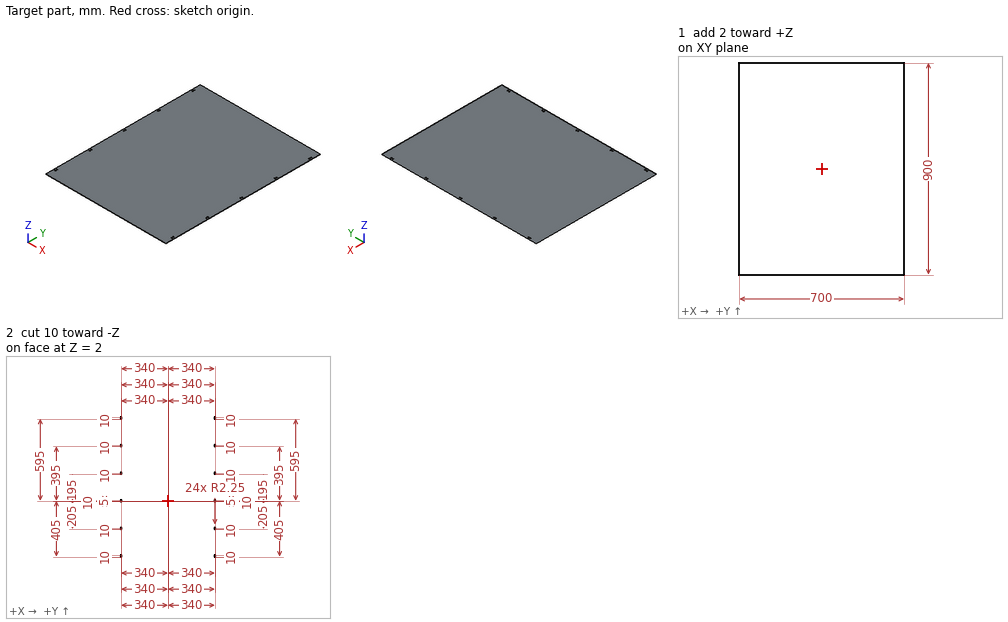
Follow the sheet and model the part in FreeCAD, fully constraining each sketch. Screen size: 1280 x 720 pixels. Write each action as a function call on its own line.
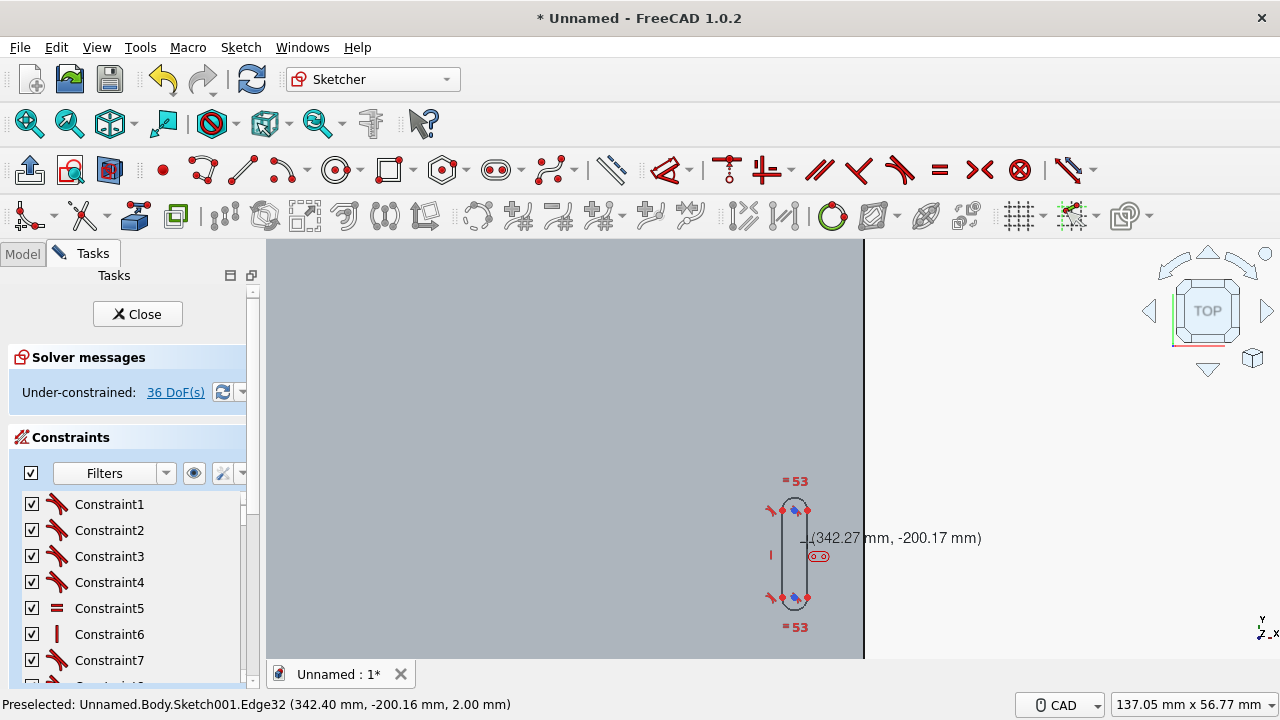
scroll(808, 539, down, 16)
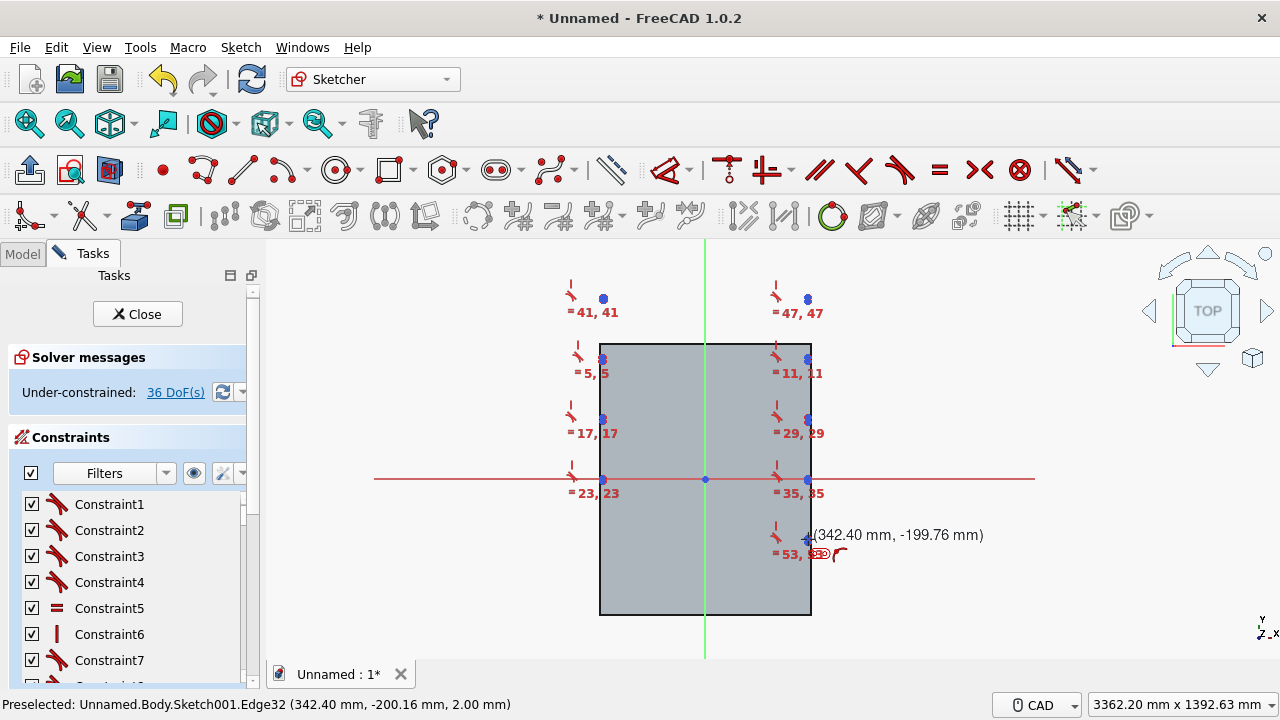
scroll(603, 541, up, 18)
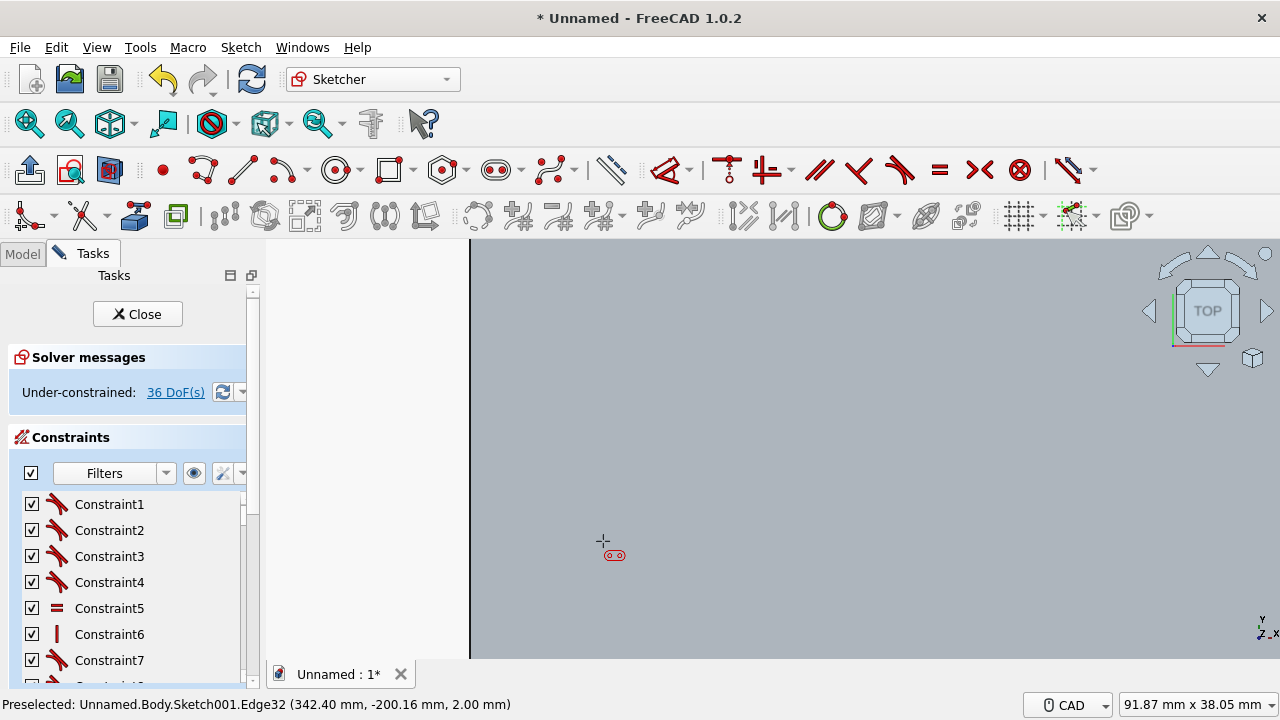
scroll(603, 541, down, 18)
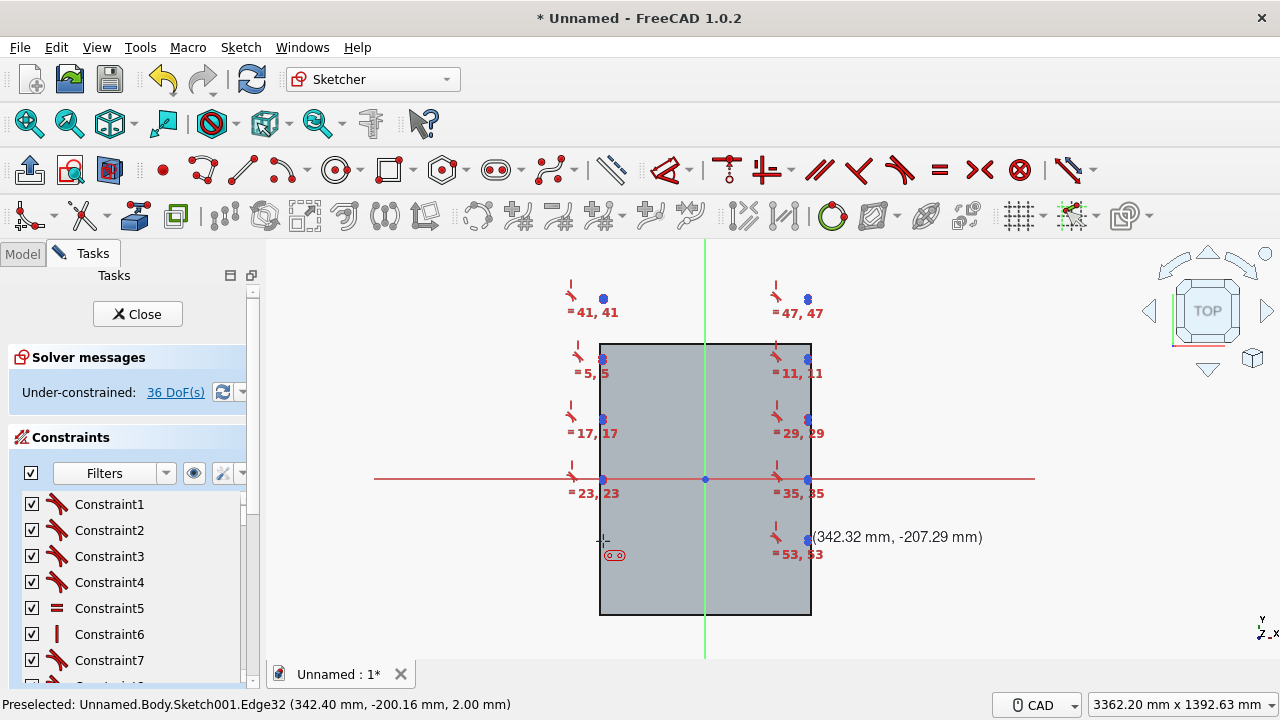
click(603, 541)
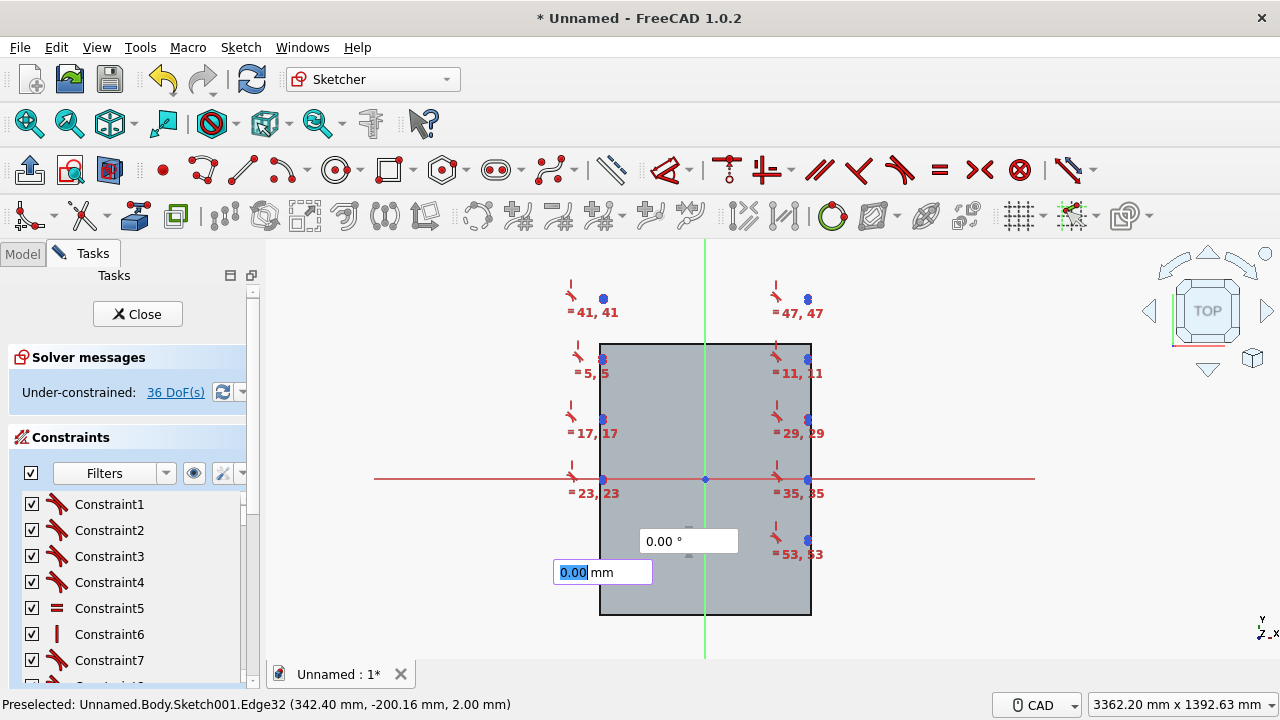
scroll(603, 538, up, 9)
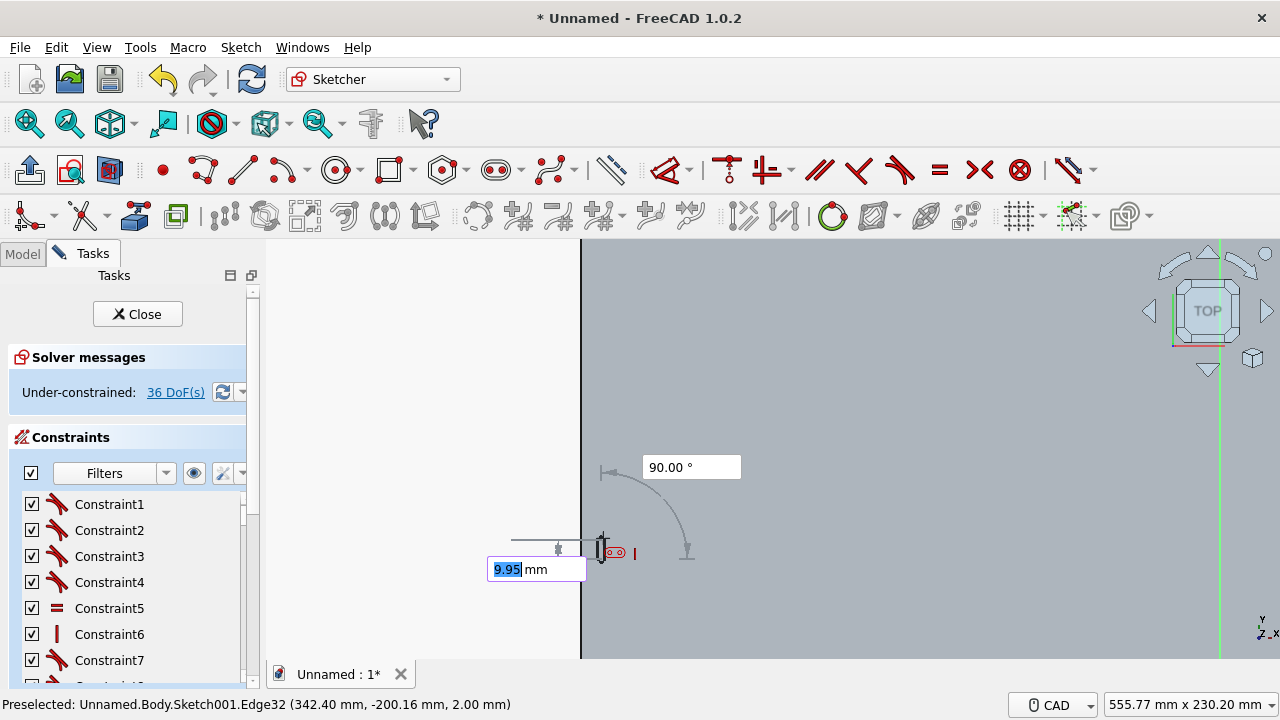
click(601, 536)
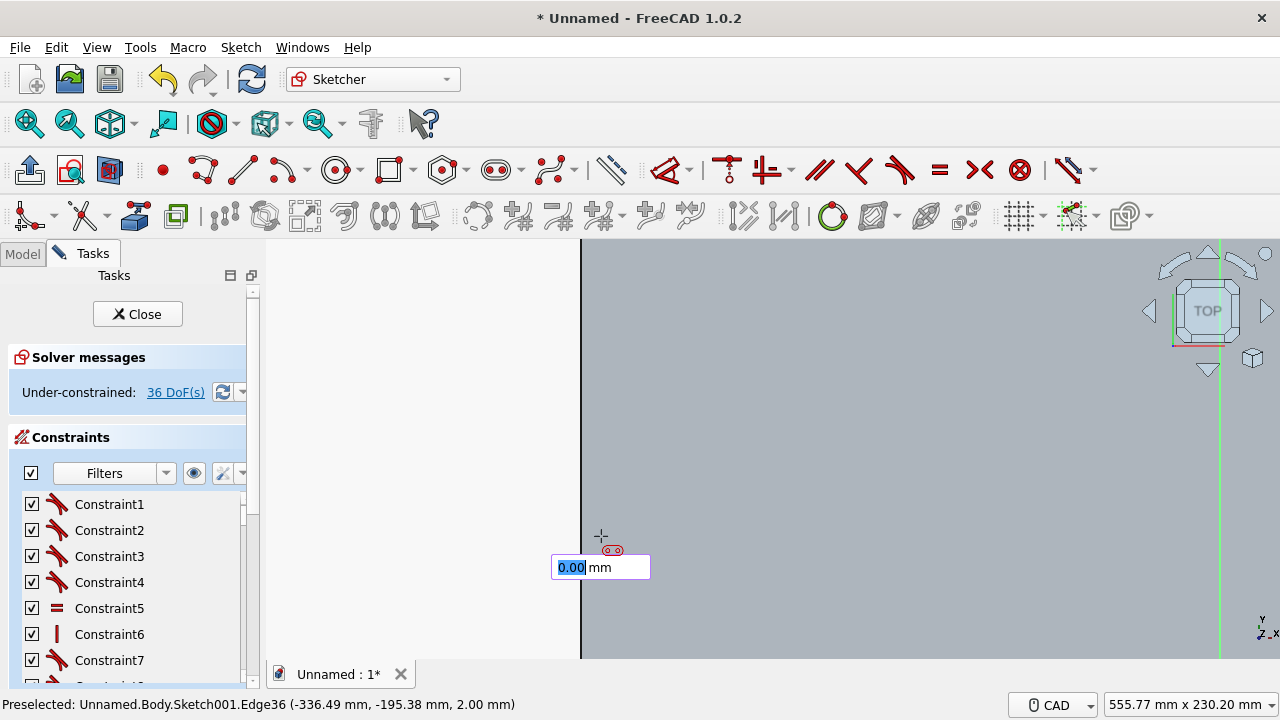
scroll(595, 545, up, 7)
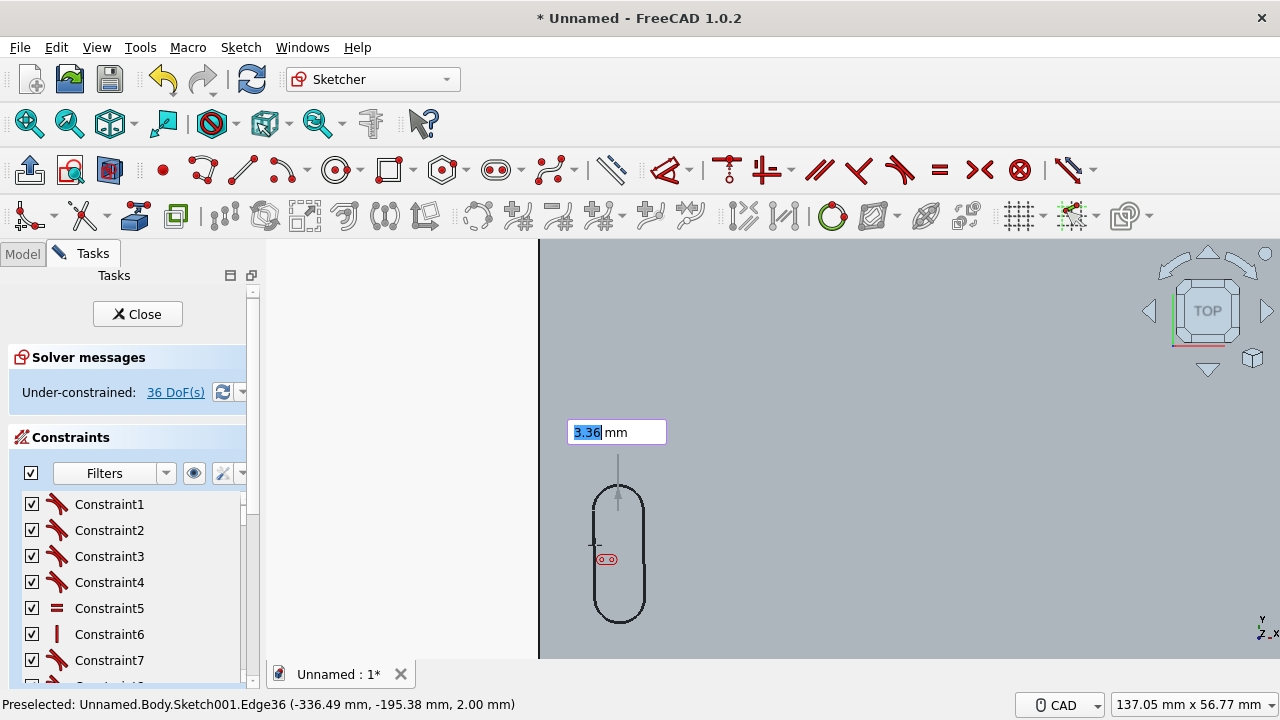
click(596, 544)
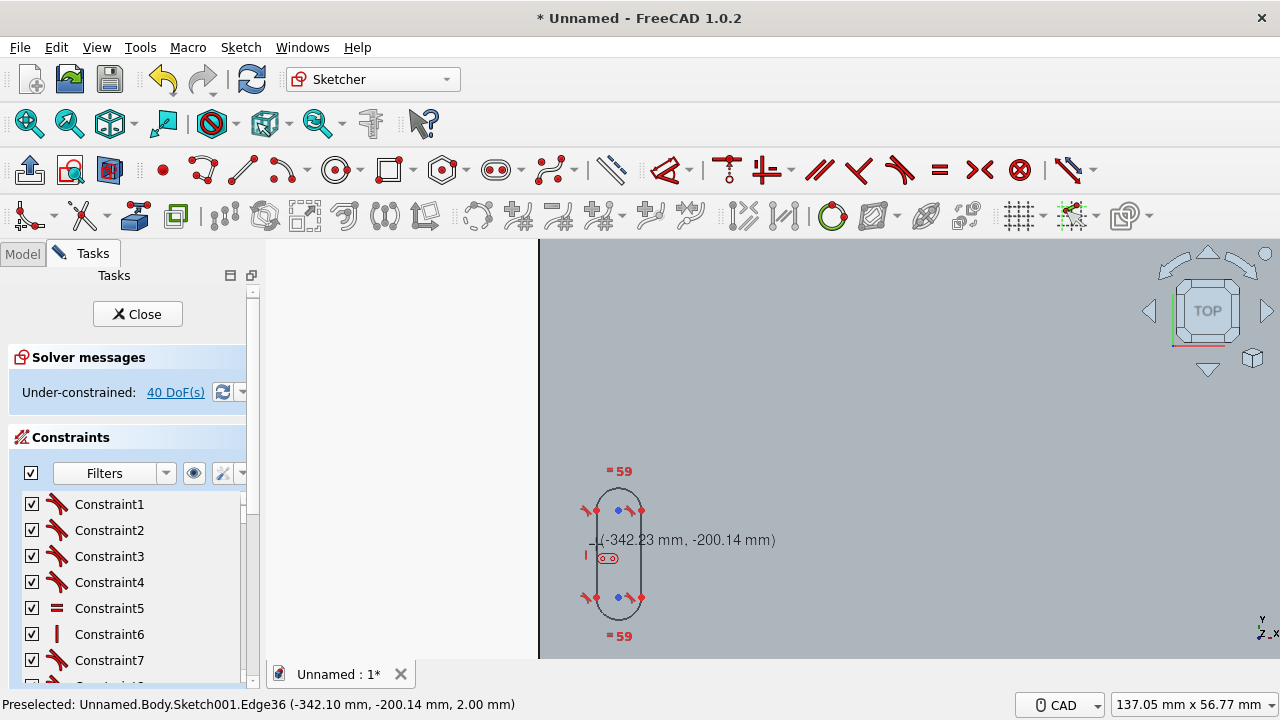
scroll(602, 539, down, 16)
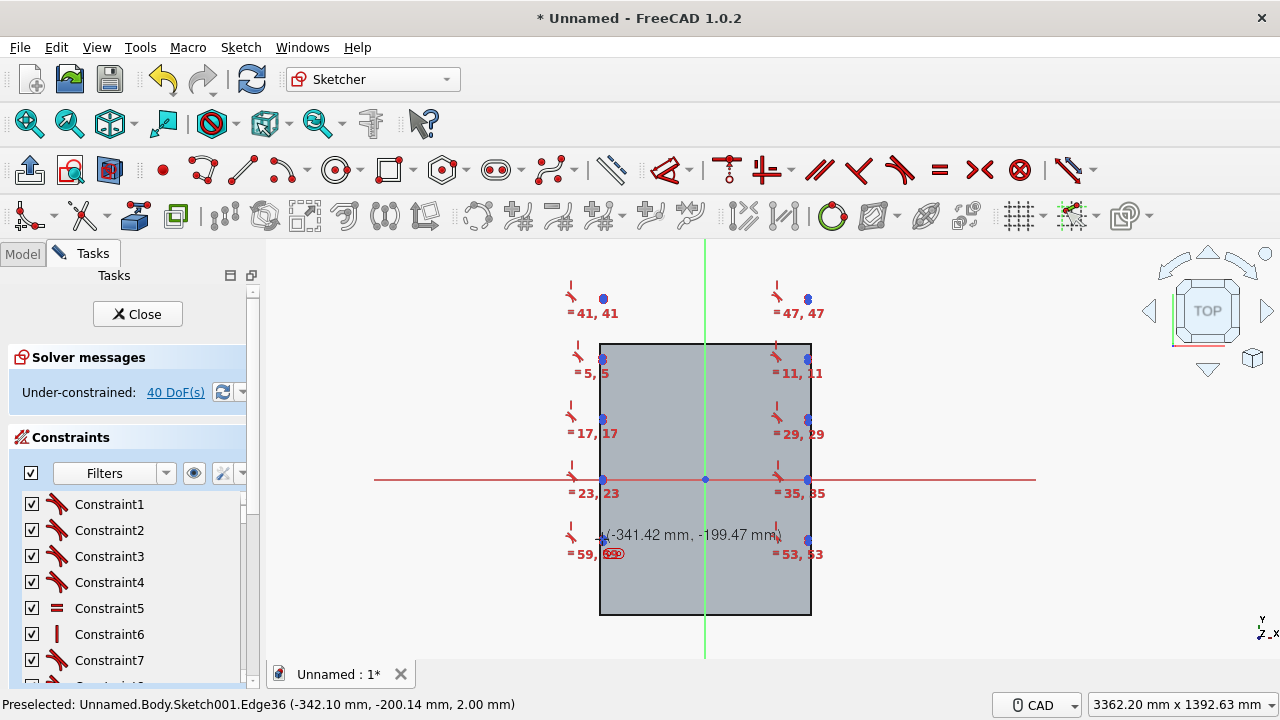
scroll(808, 602, up, 18)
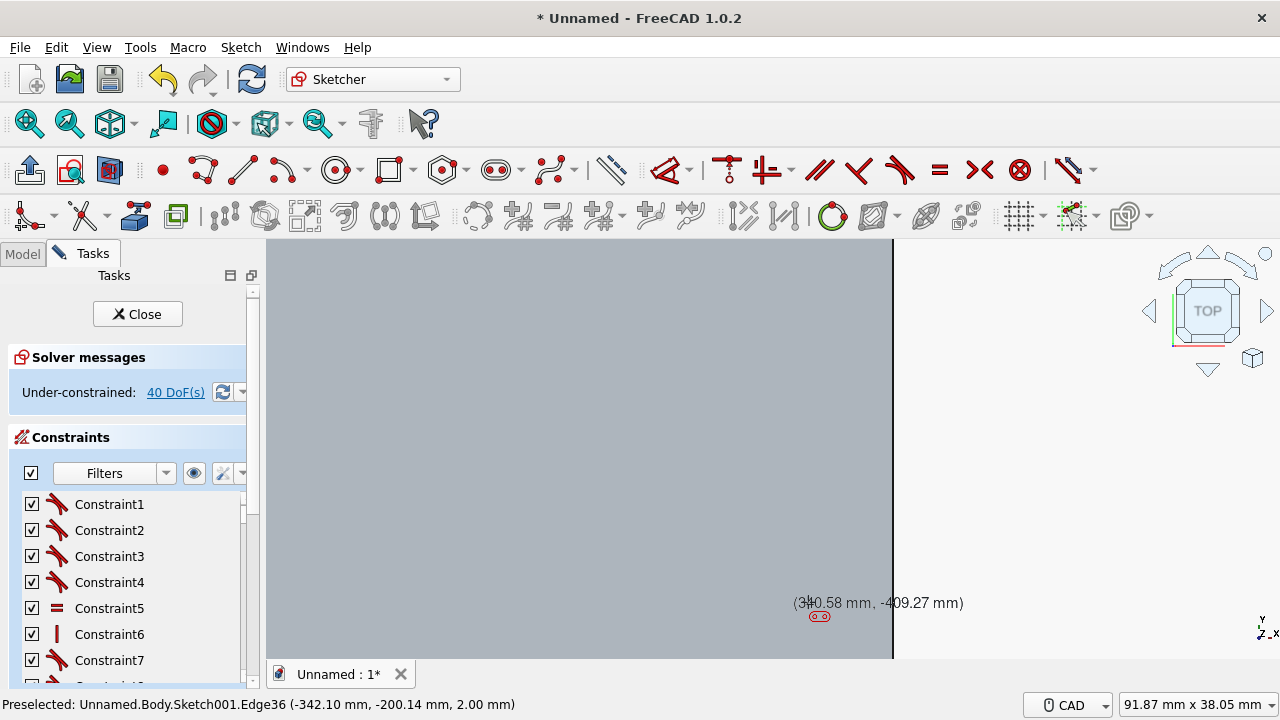
scroll(808, 602, down, 18)